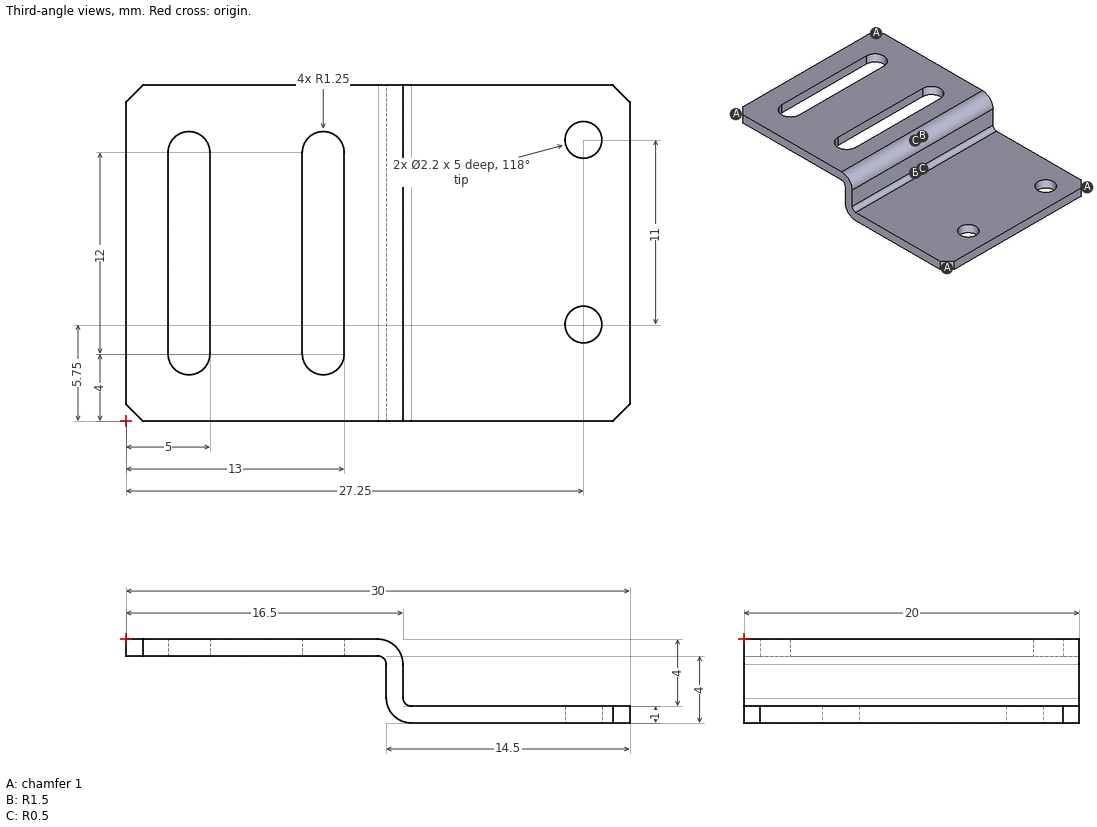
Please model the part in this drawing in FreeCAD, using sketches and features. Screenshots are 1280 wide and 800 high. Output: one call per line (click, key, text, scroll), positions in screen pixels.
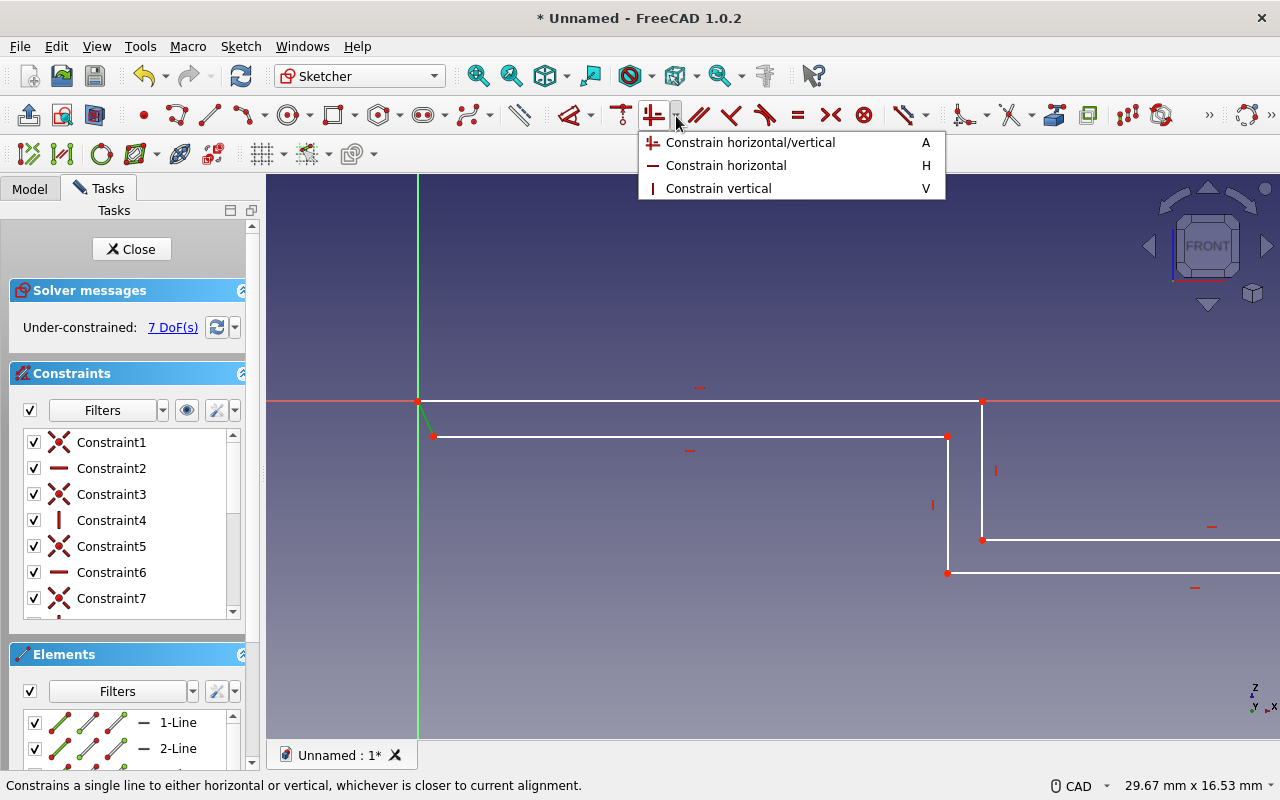
click(792, 188)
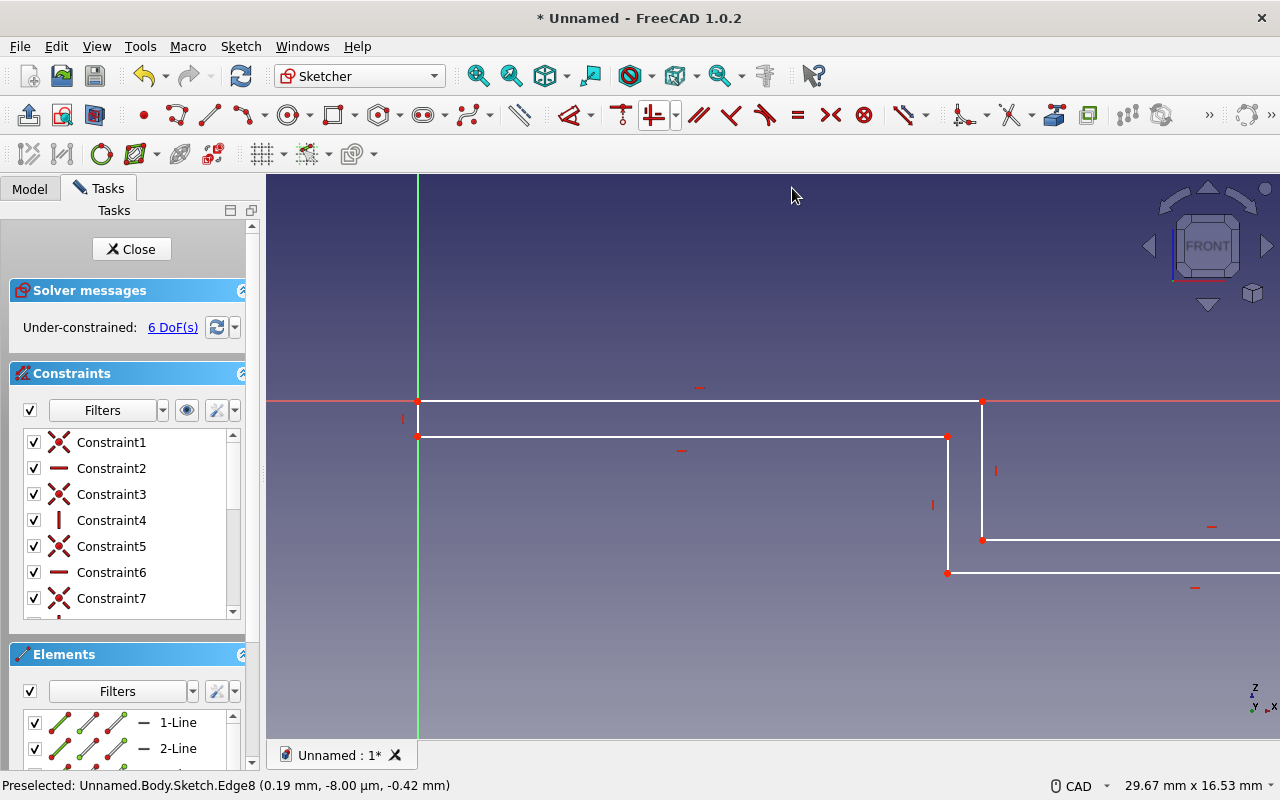
click(568, 116)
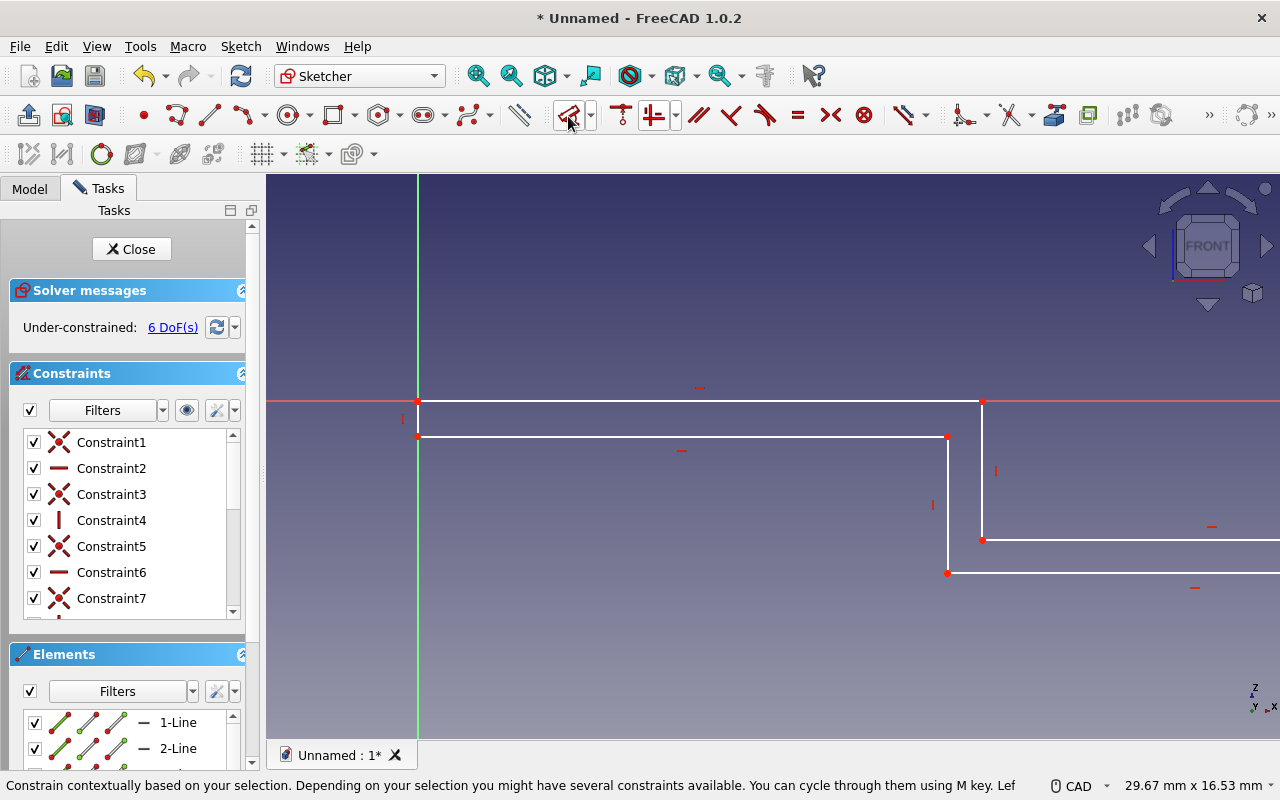
click(982, 443)
click(1016, 471)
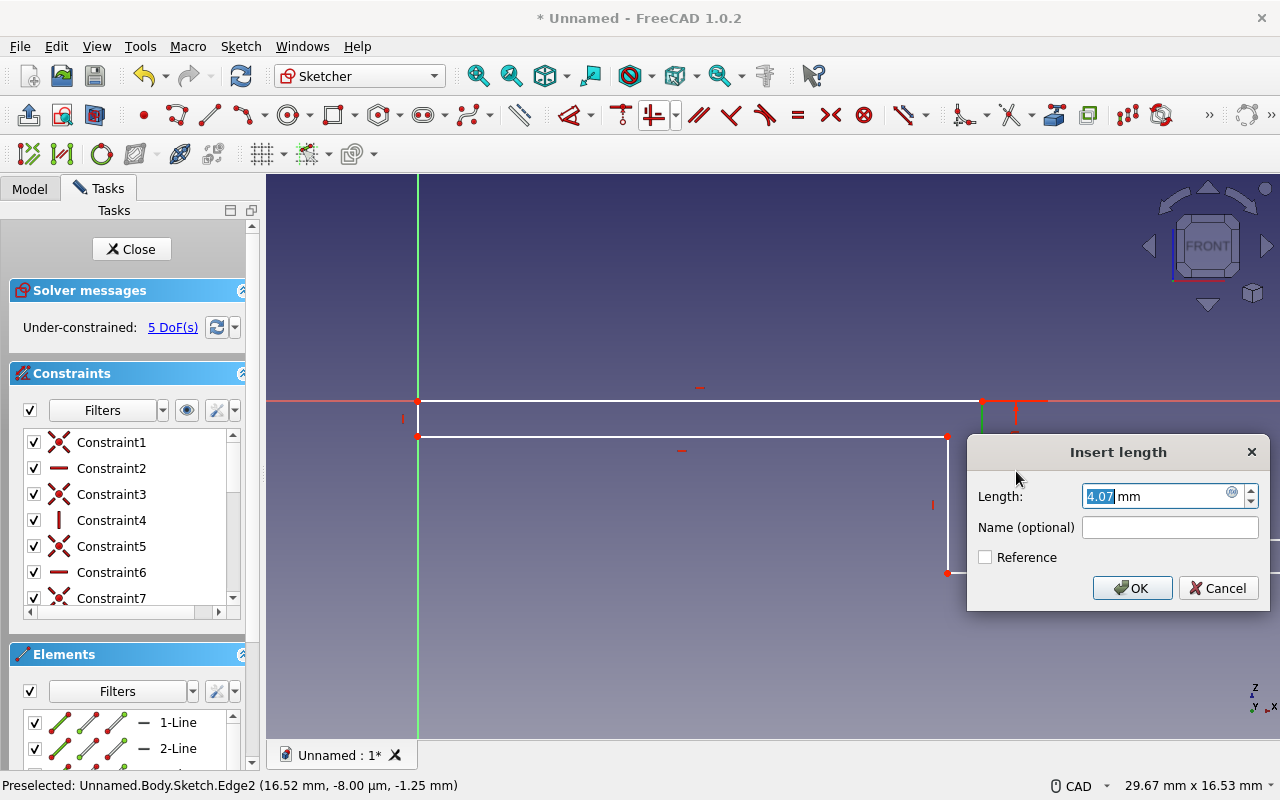
text(4)
key(Return)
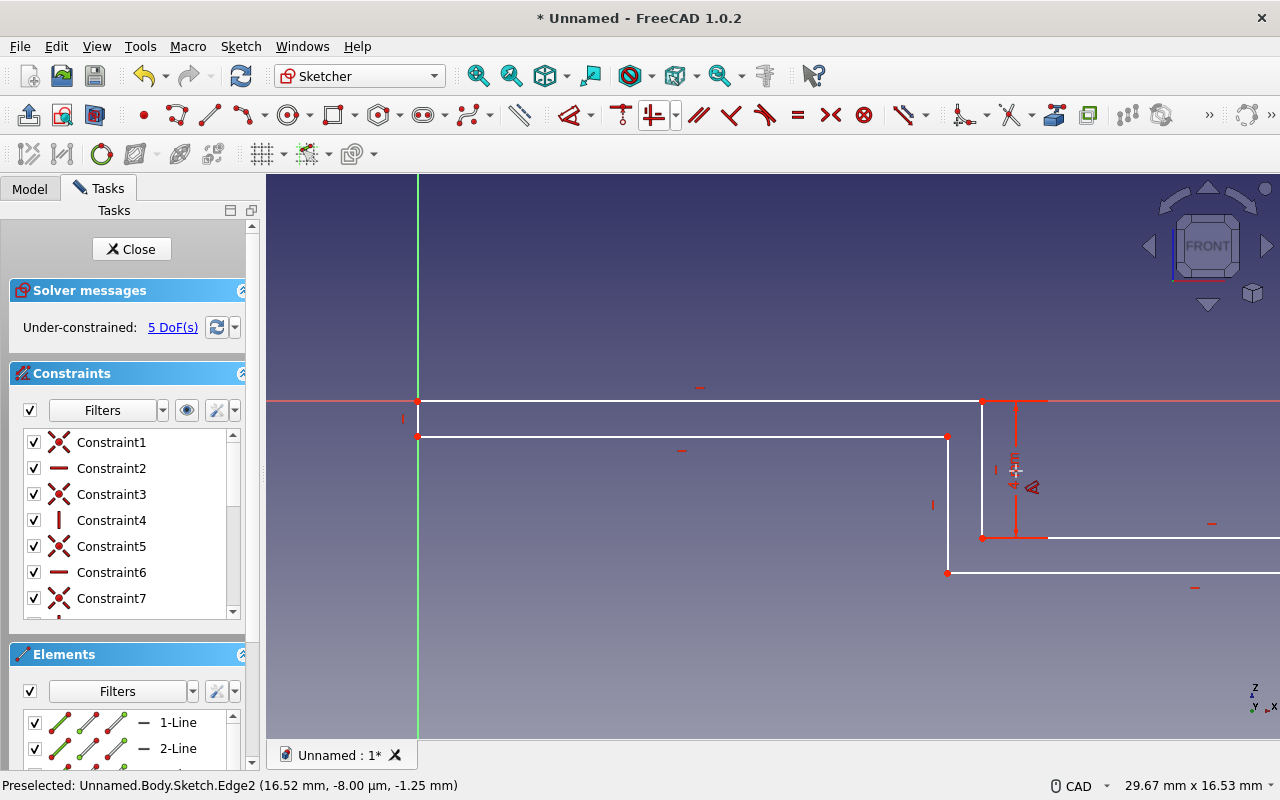
scroll(430, 420, down, 3)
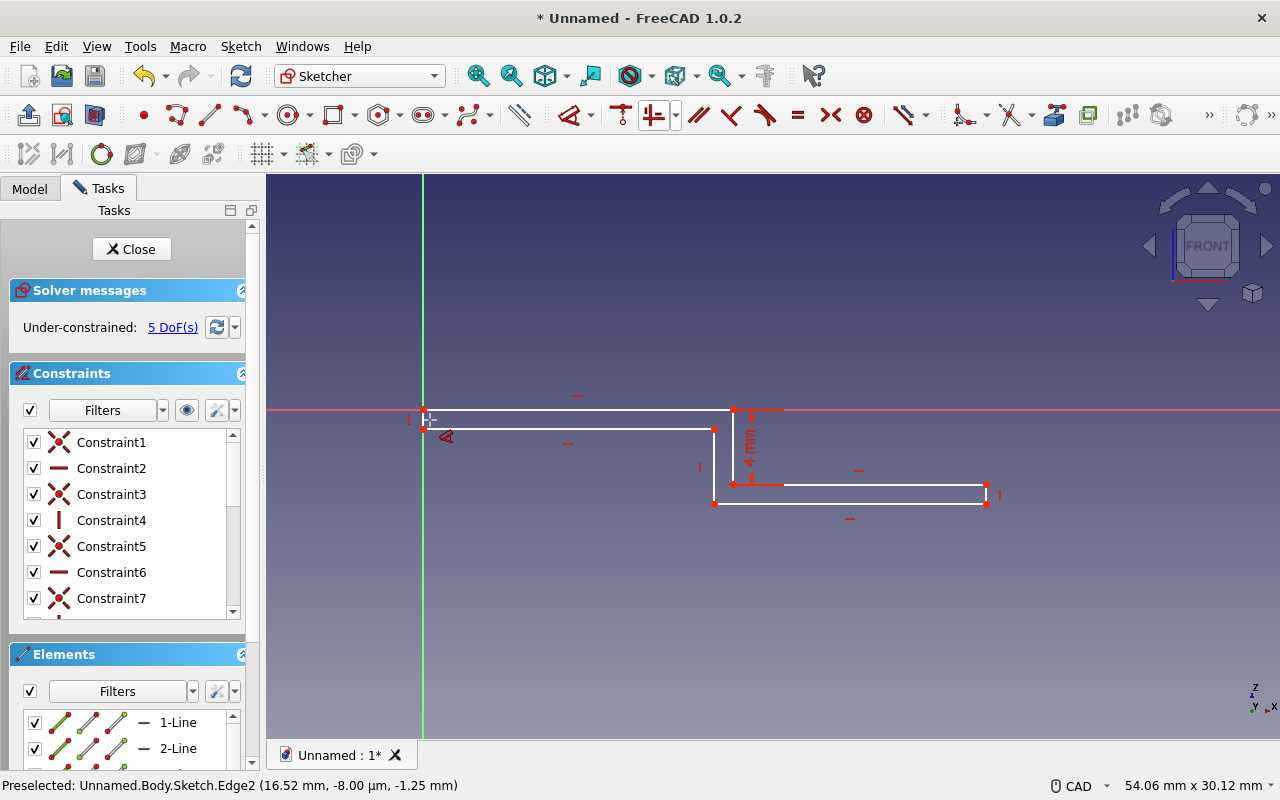
scroll(986, 491, up, 5)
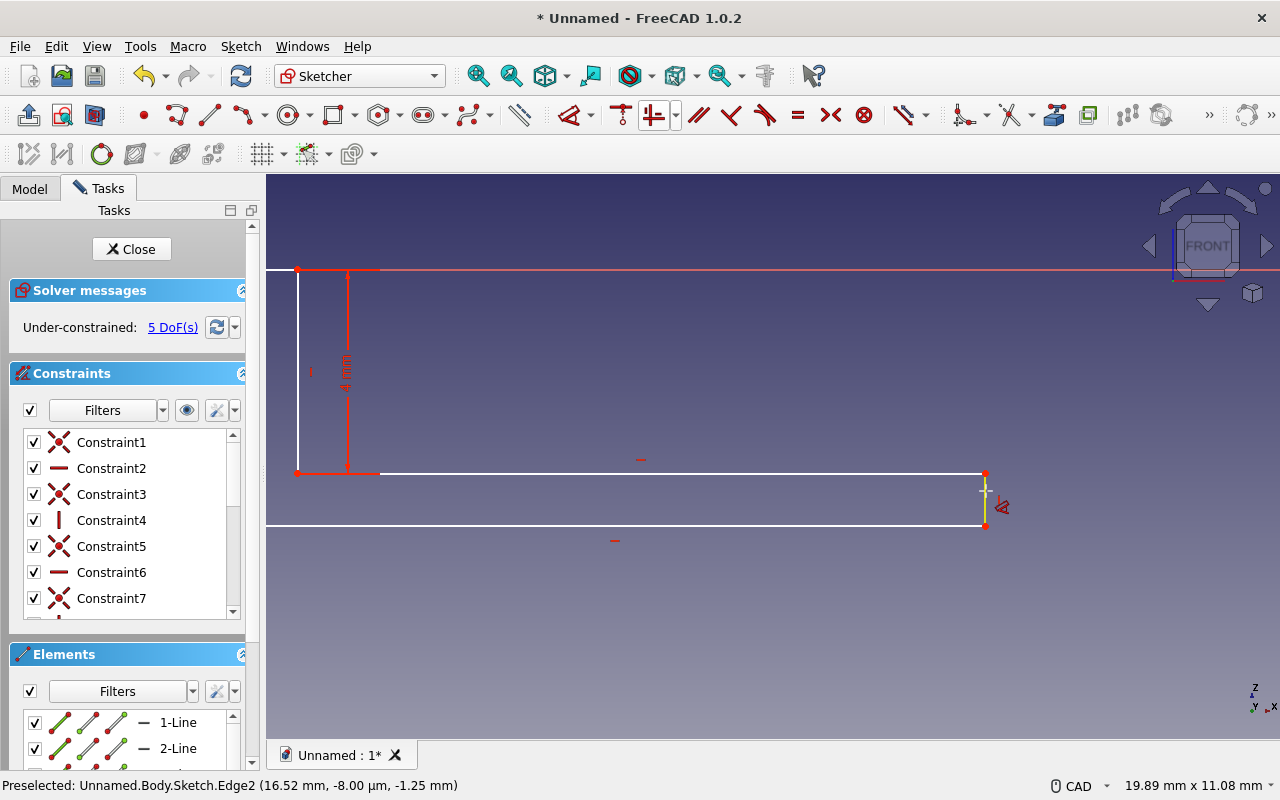
click(985, 489)
click(1019, 500)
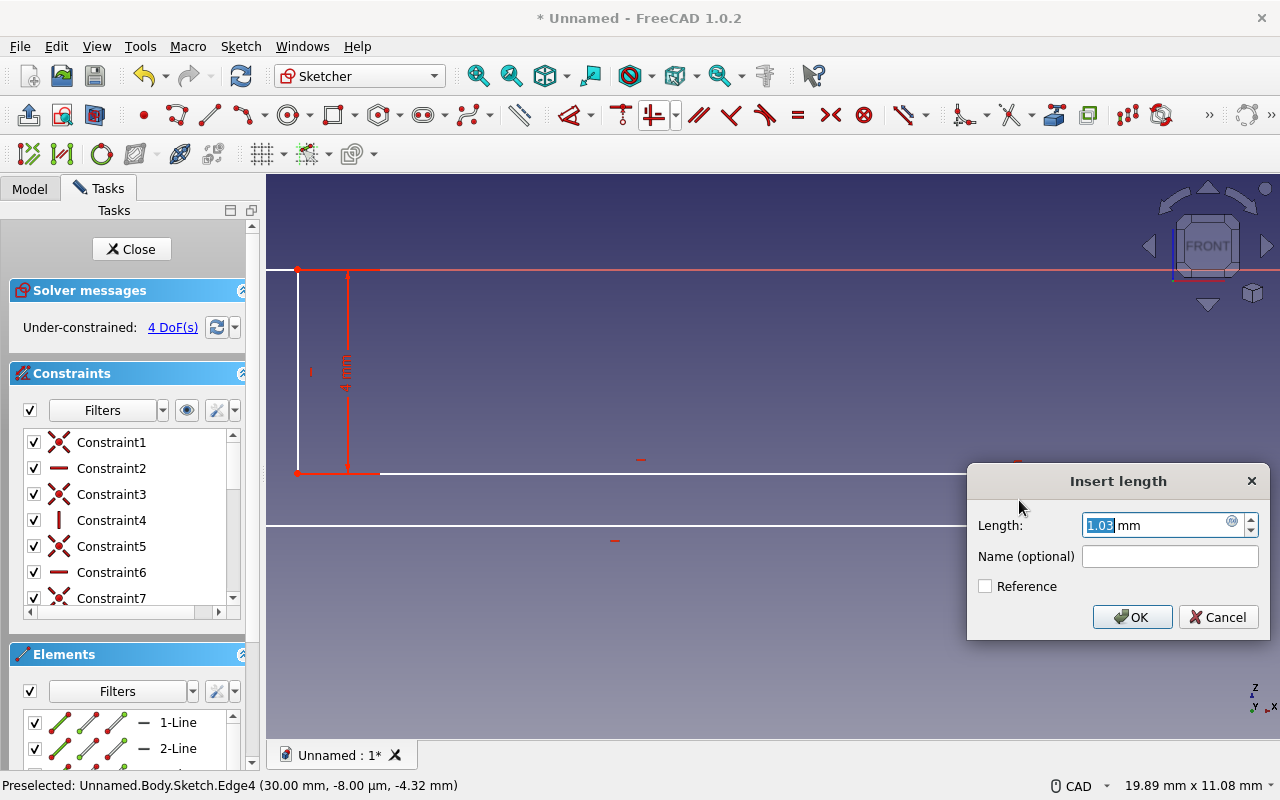
text(1)
key(Return)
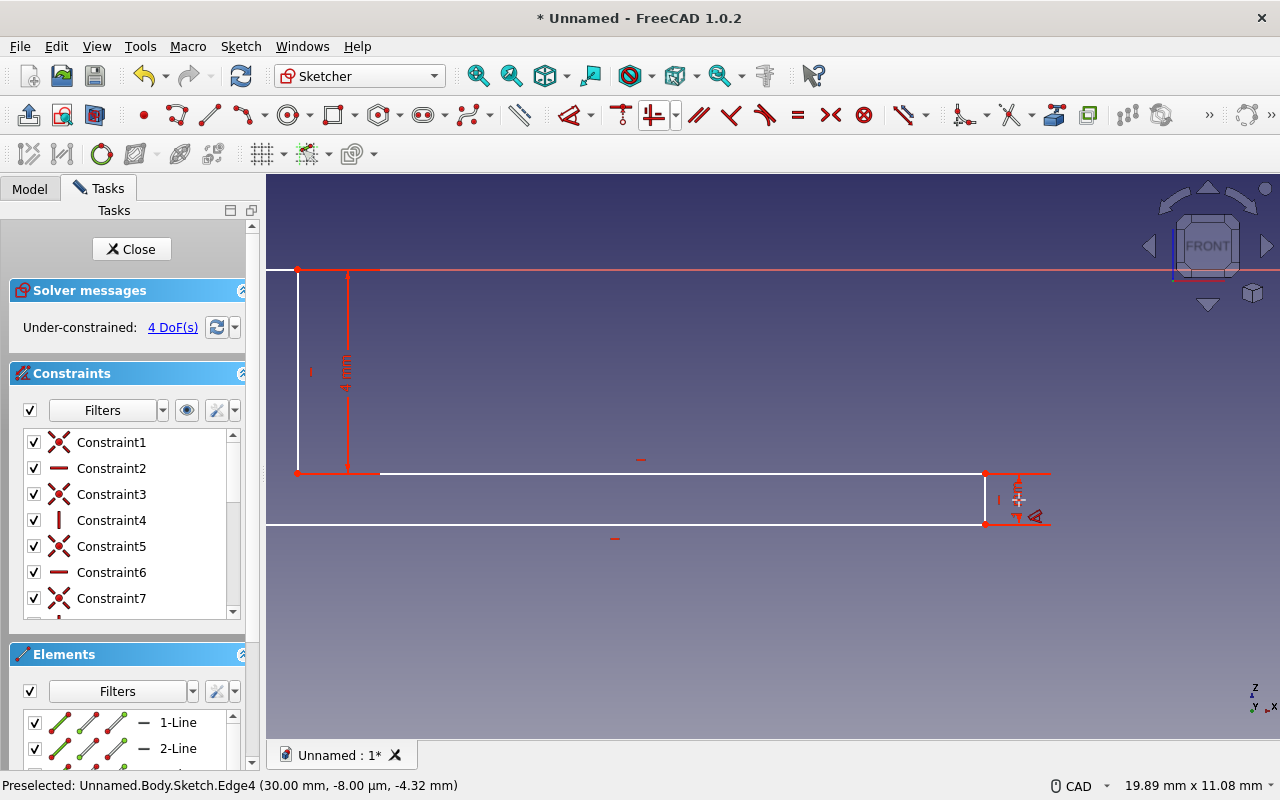
scroll(986, 491, down, 5)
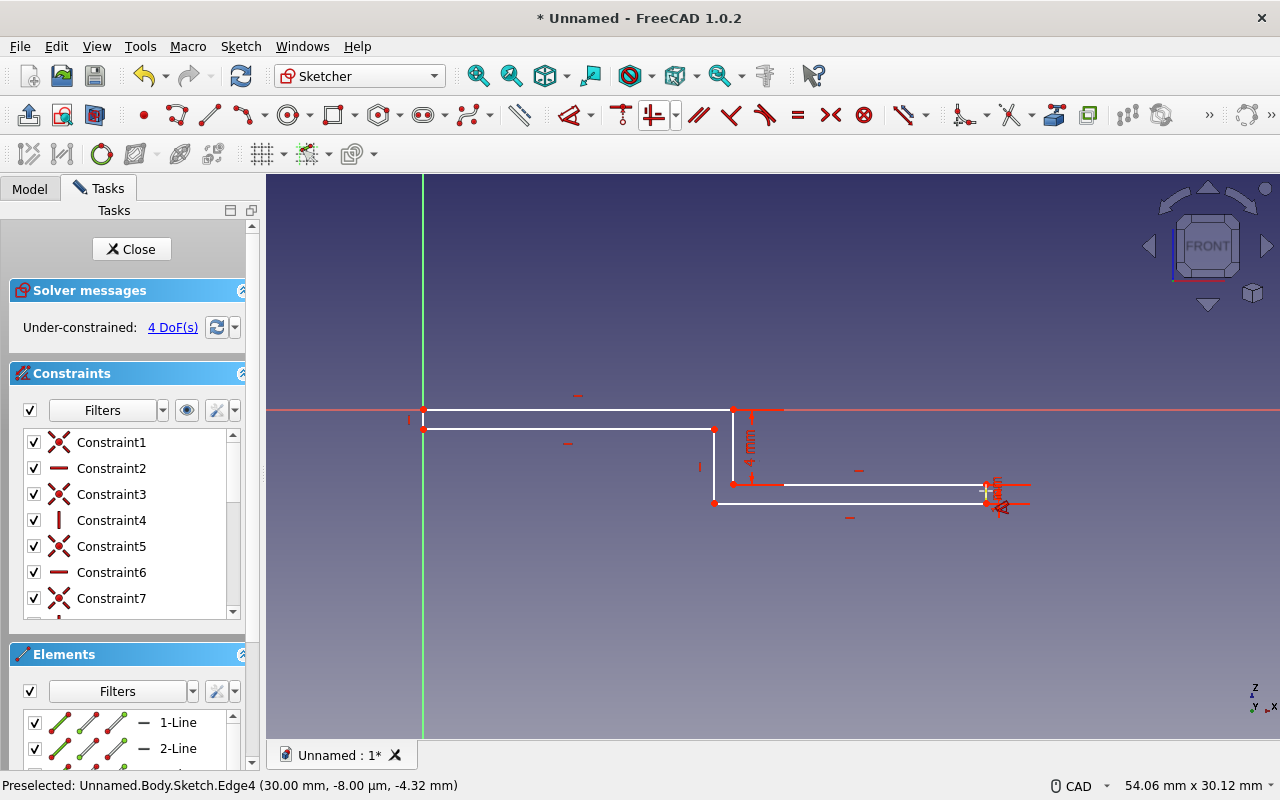
click(714, 481)
click(680, 467)